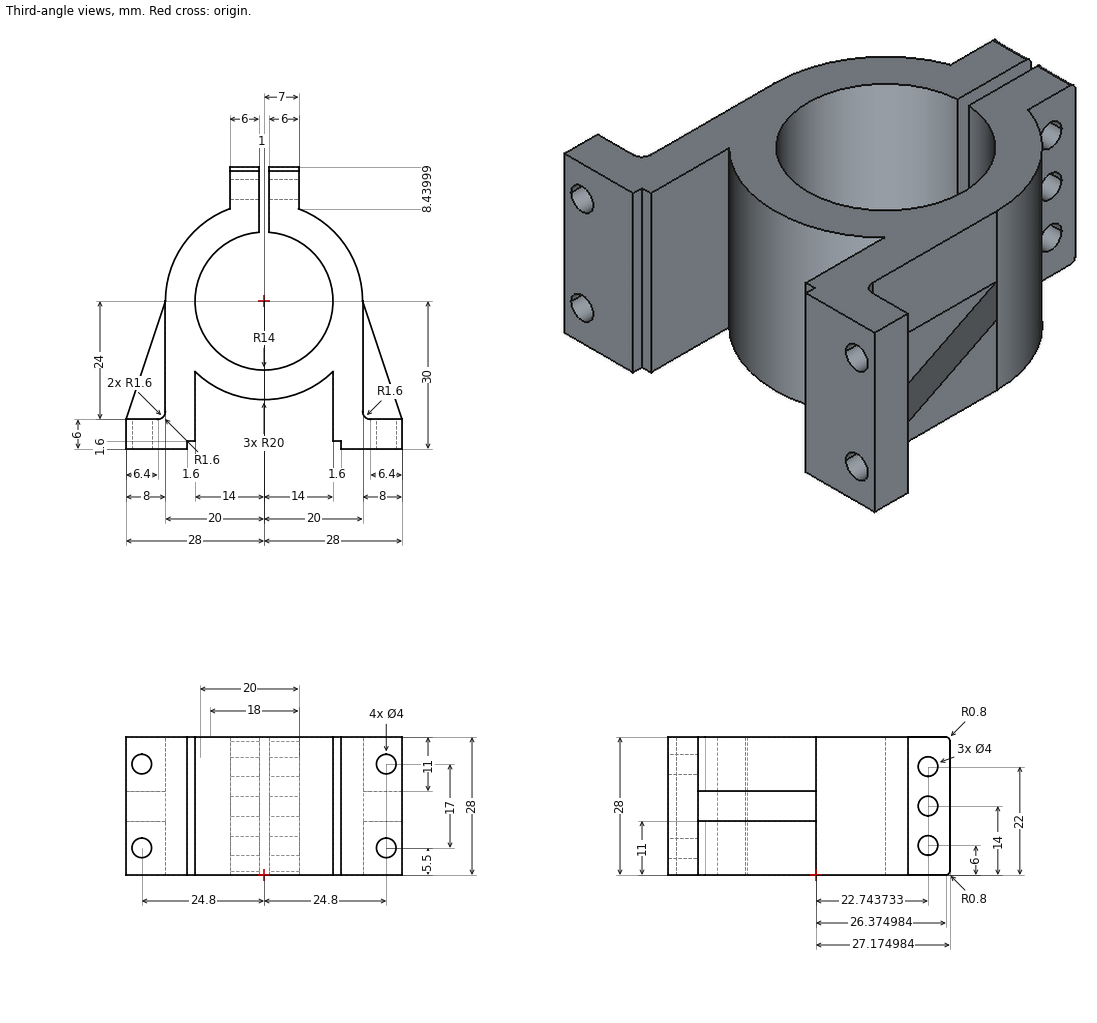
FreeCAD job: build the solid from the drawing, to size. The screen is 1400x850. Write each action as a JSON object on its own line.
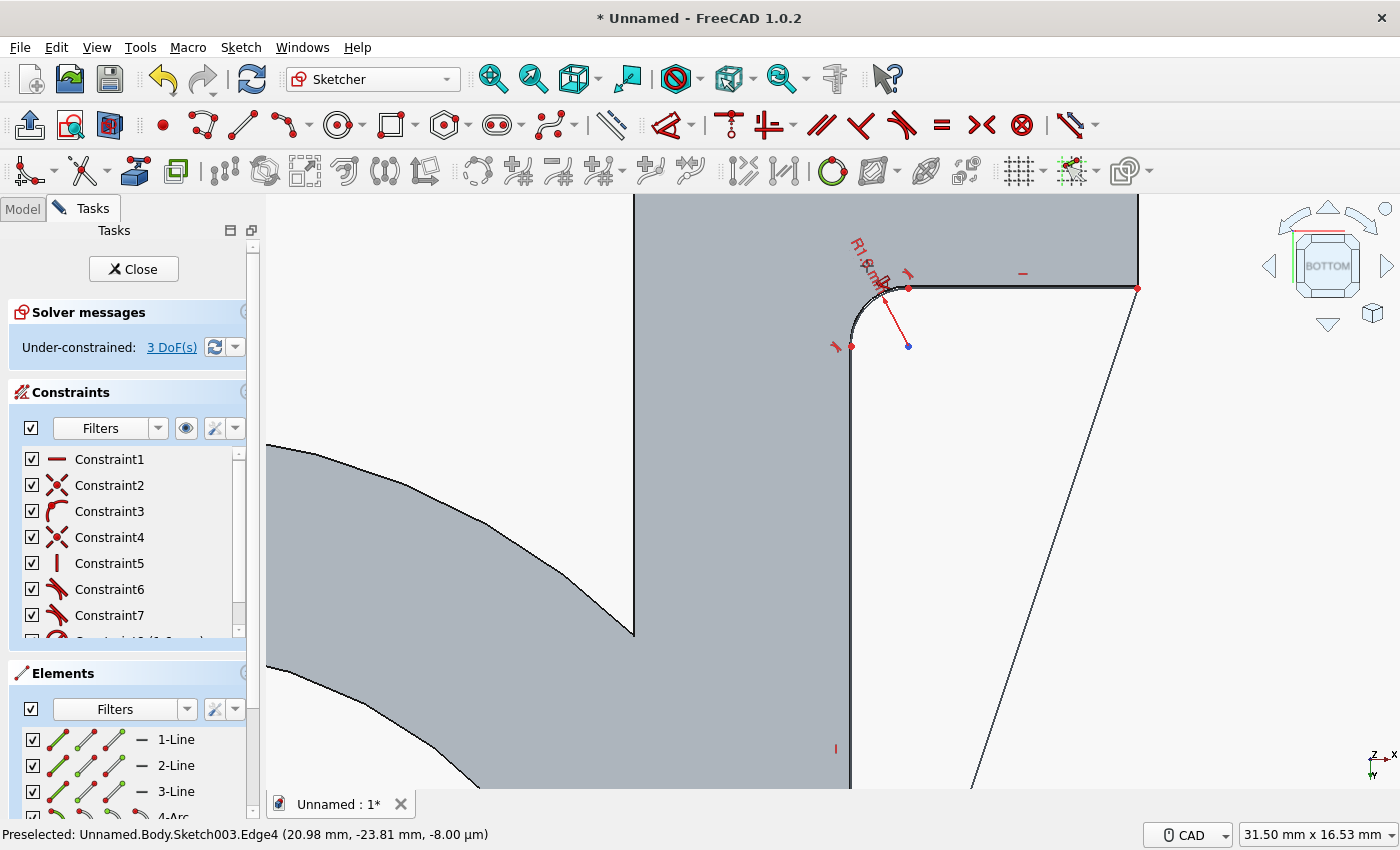
{"action": "left_click", "coordinate": [1052, 547]}
{"action": "left_click", "coordinate": [994, 254]}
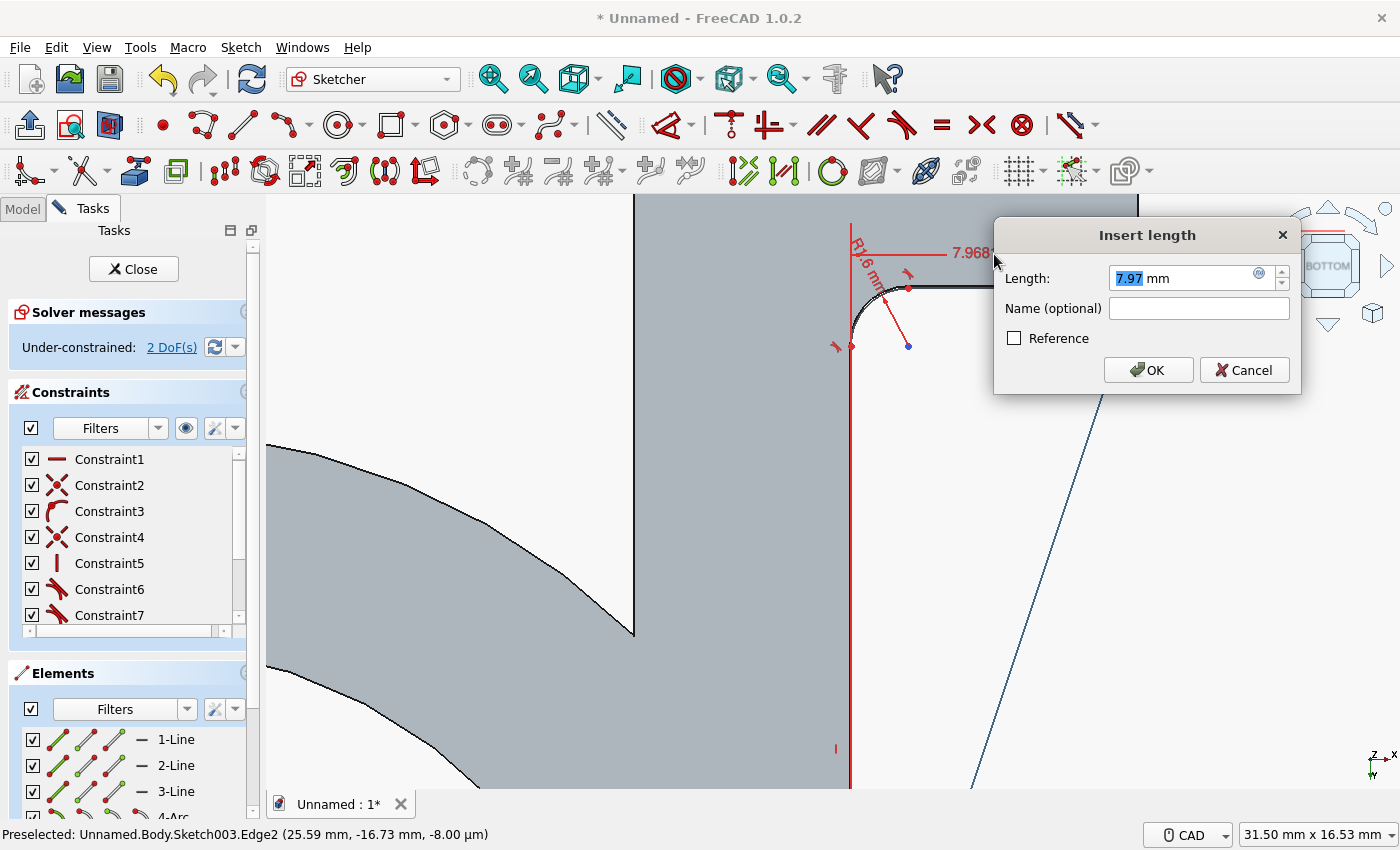
{"action": "type", "text": "8"}
{"action": "key", "text": "Return"}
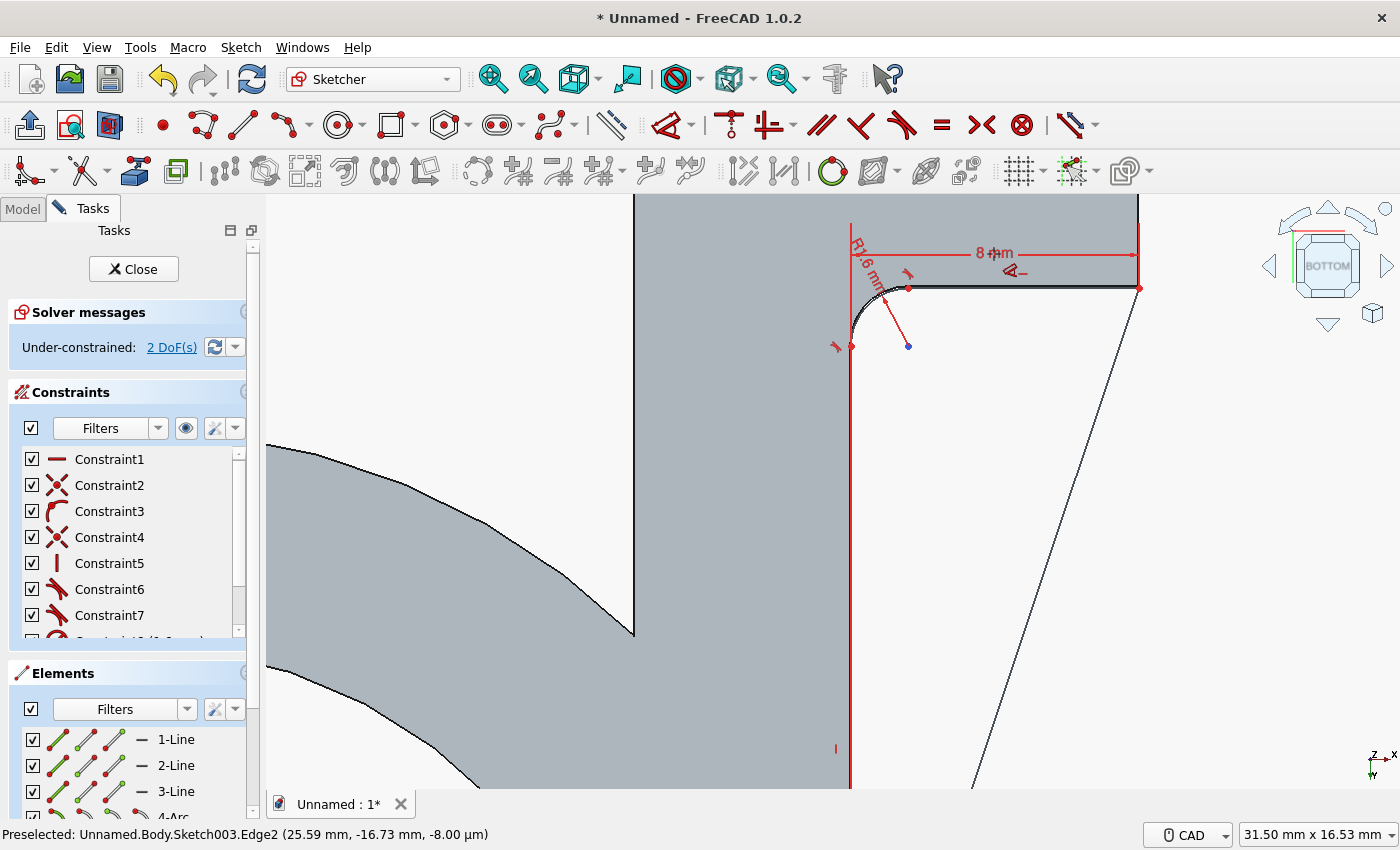
{"action": "left_click", "coordinate": [909, 288]}
{"action": "left_click", "coordinate": [943, 525]}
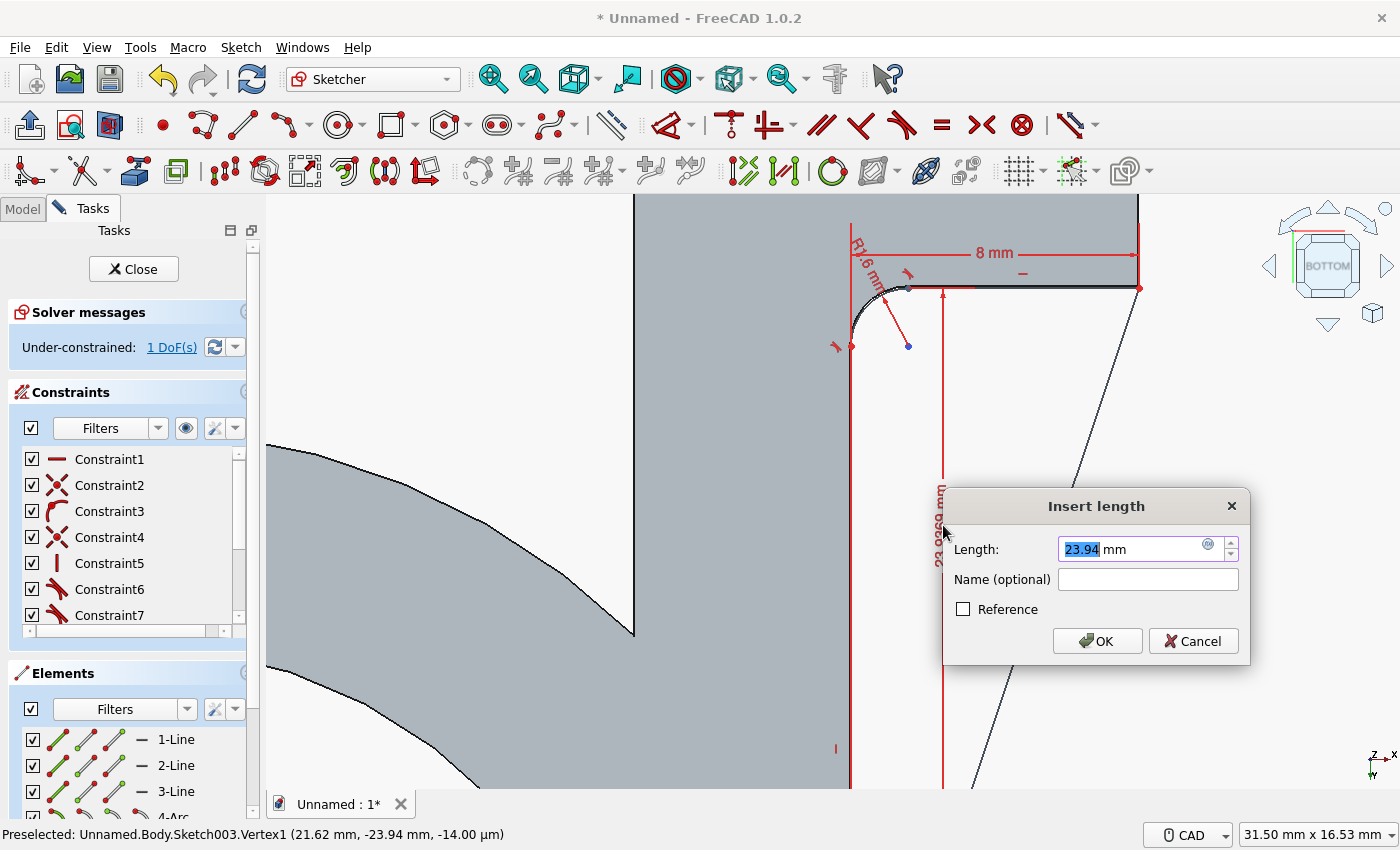
{"action": "type", "text": "24"}
{"action": "key", "text": "Return"}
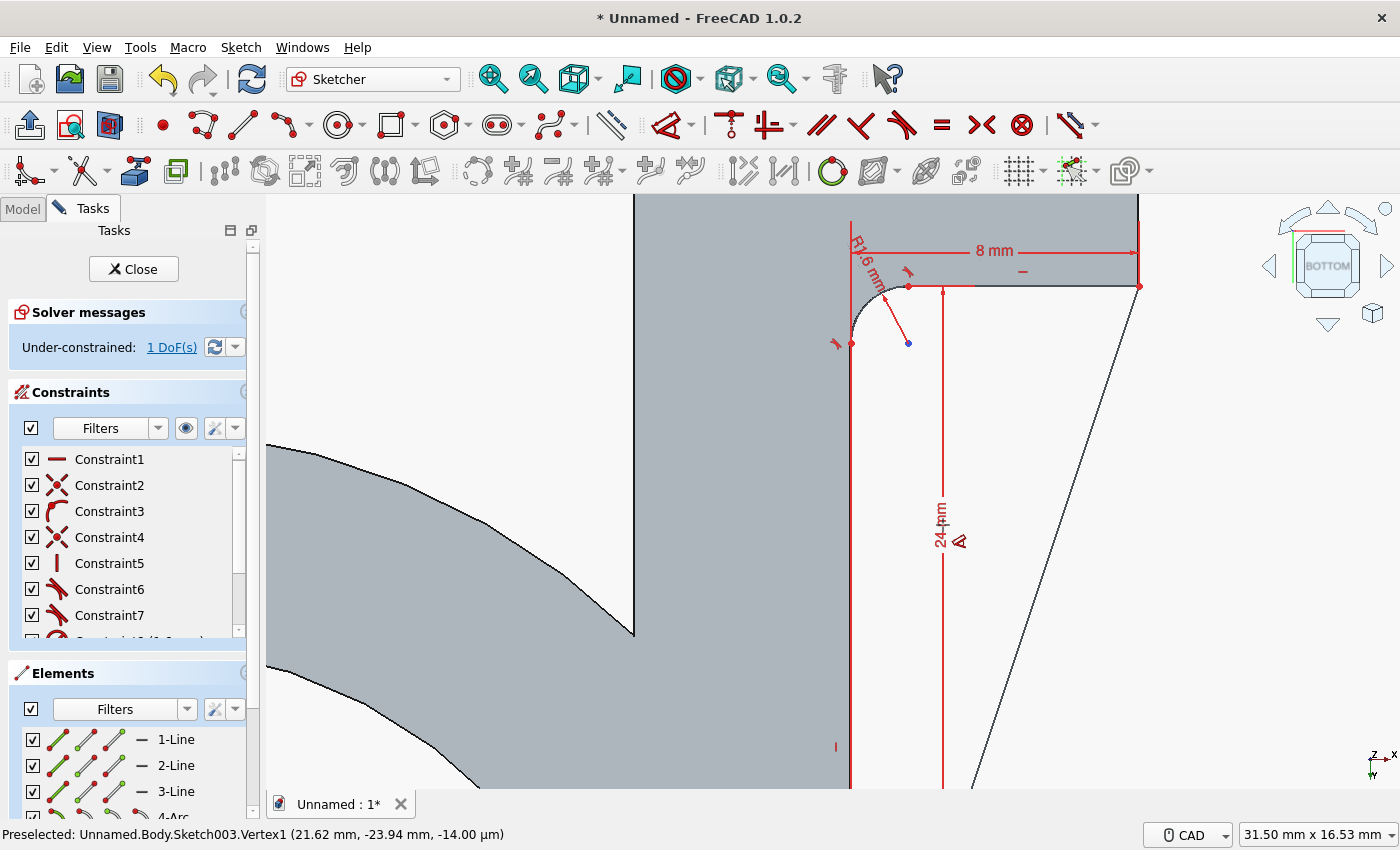
{"action": "left_click", "coordinate": [1139, 286]}
{"action": "left_click", "coordinate": [717, 252]}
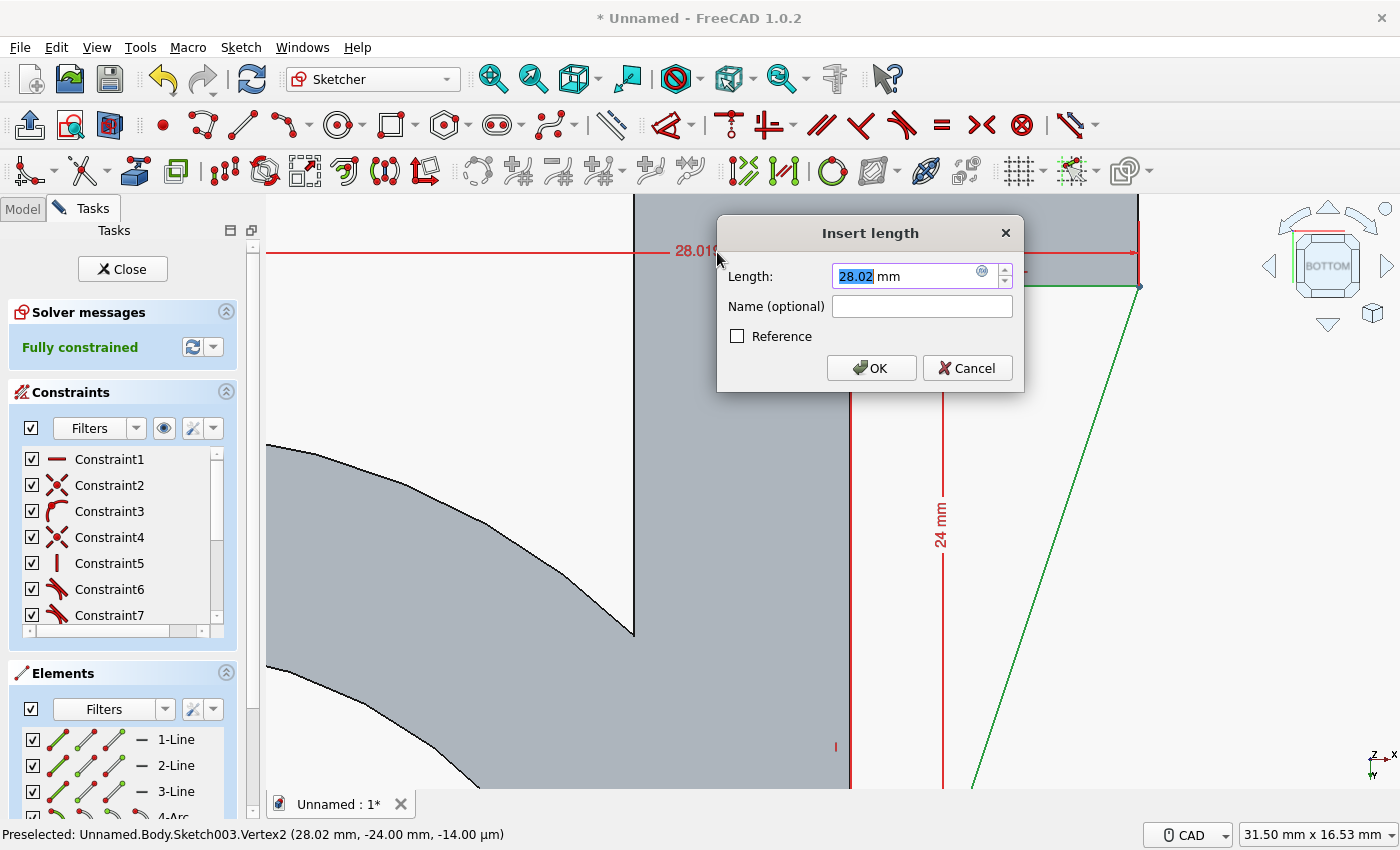
{"action": "type", "text": "28"}
{"action": "key", "text": "Return"}
{"action": "key", "text": "Escape"}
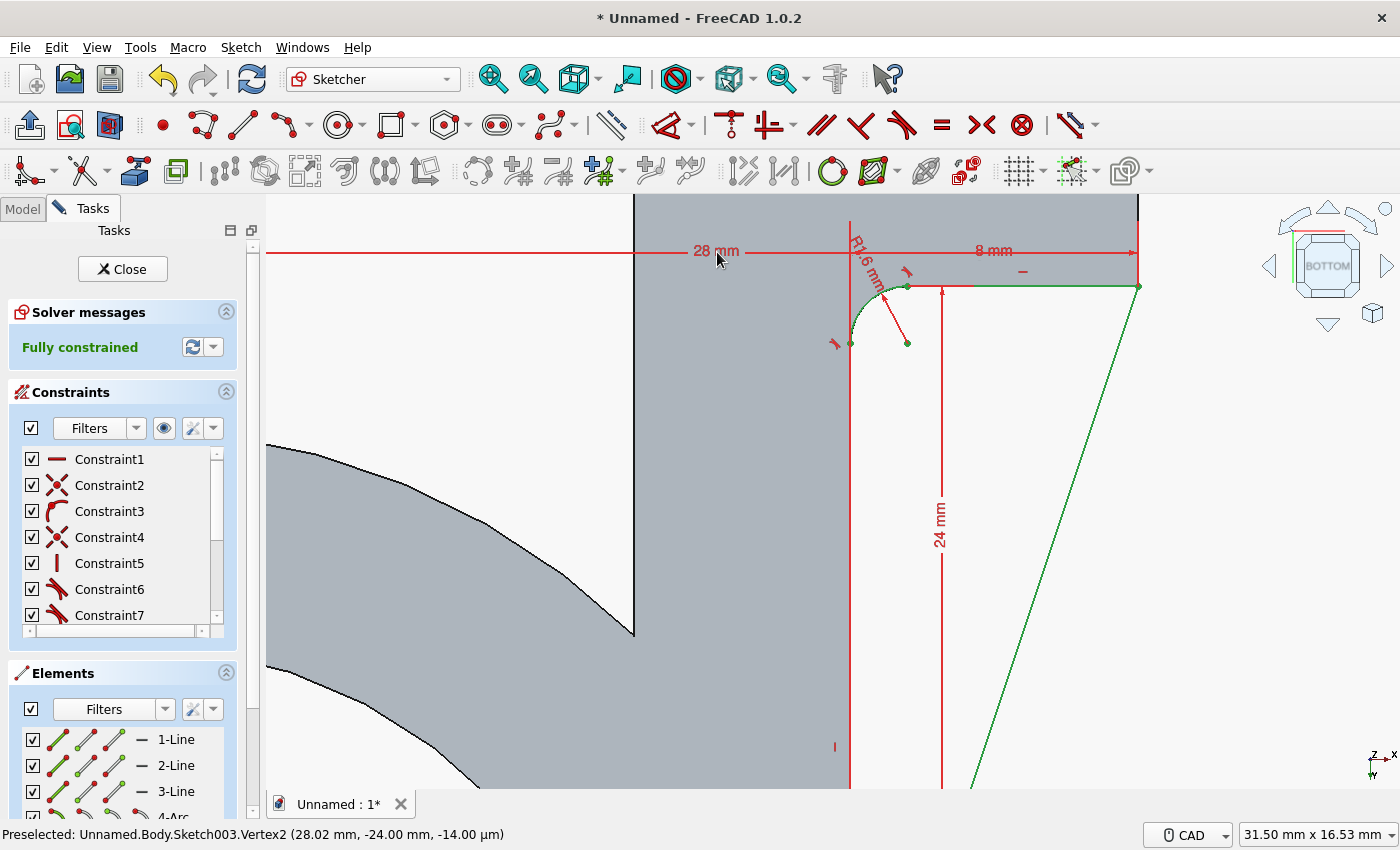
{"action": "left_click", "coordinate": [123, 269]}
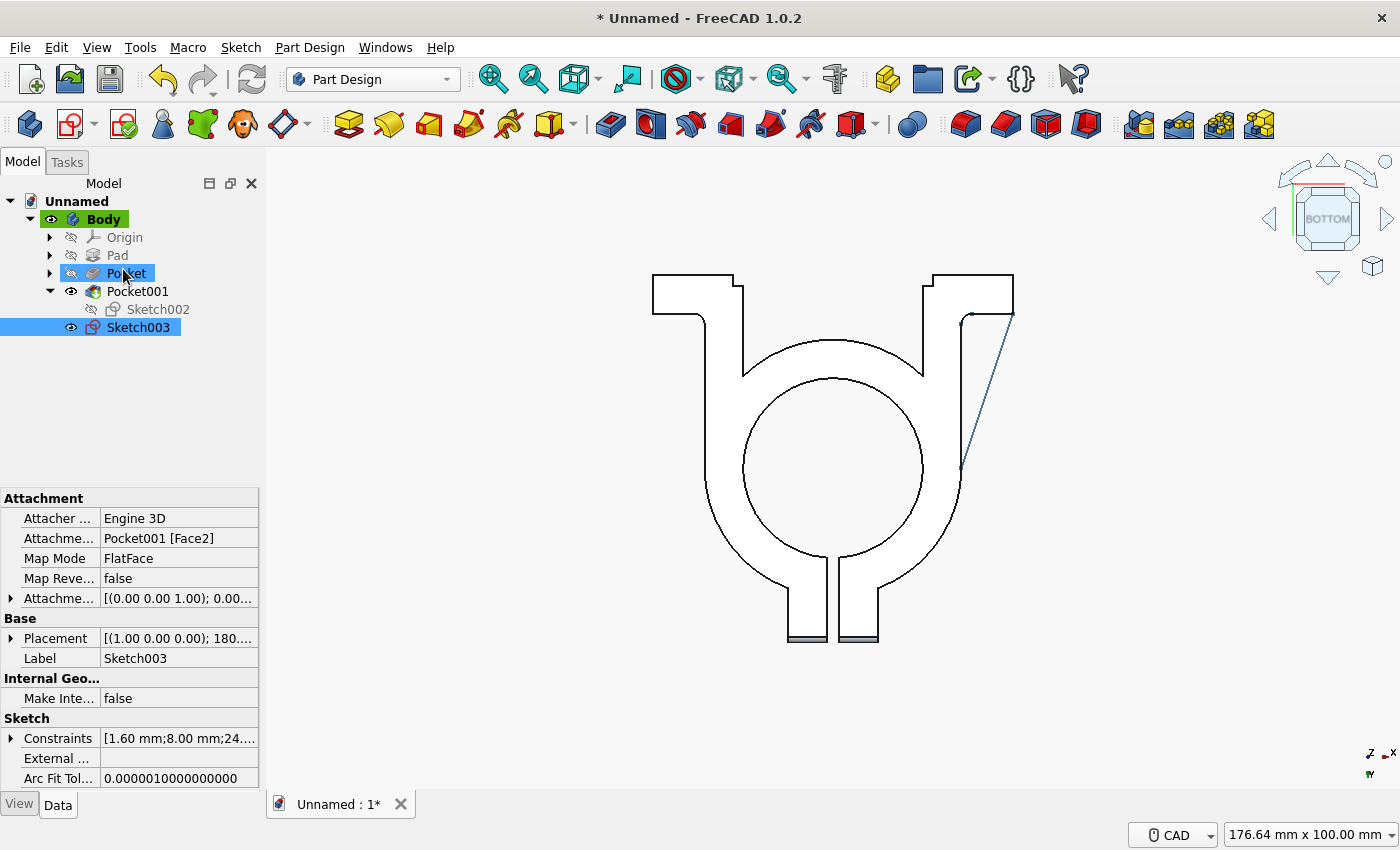
{"action": "left_click", "coordinate": [350, 124]}